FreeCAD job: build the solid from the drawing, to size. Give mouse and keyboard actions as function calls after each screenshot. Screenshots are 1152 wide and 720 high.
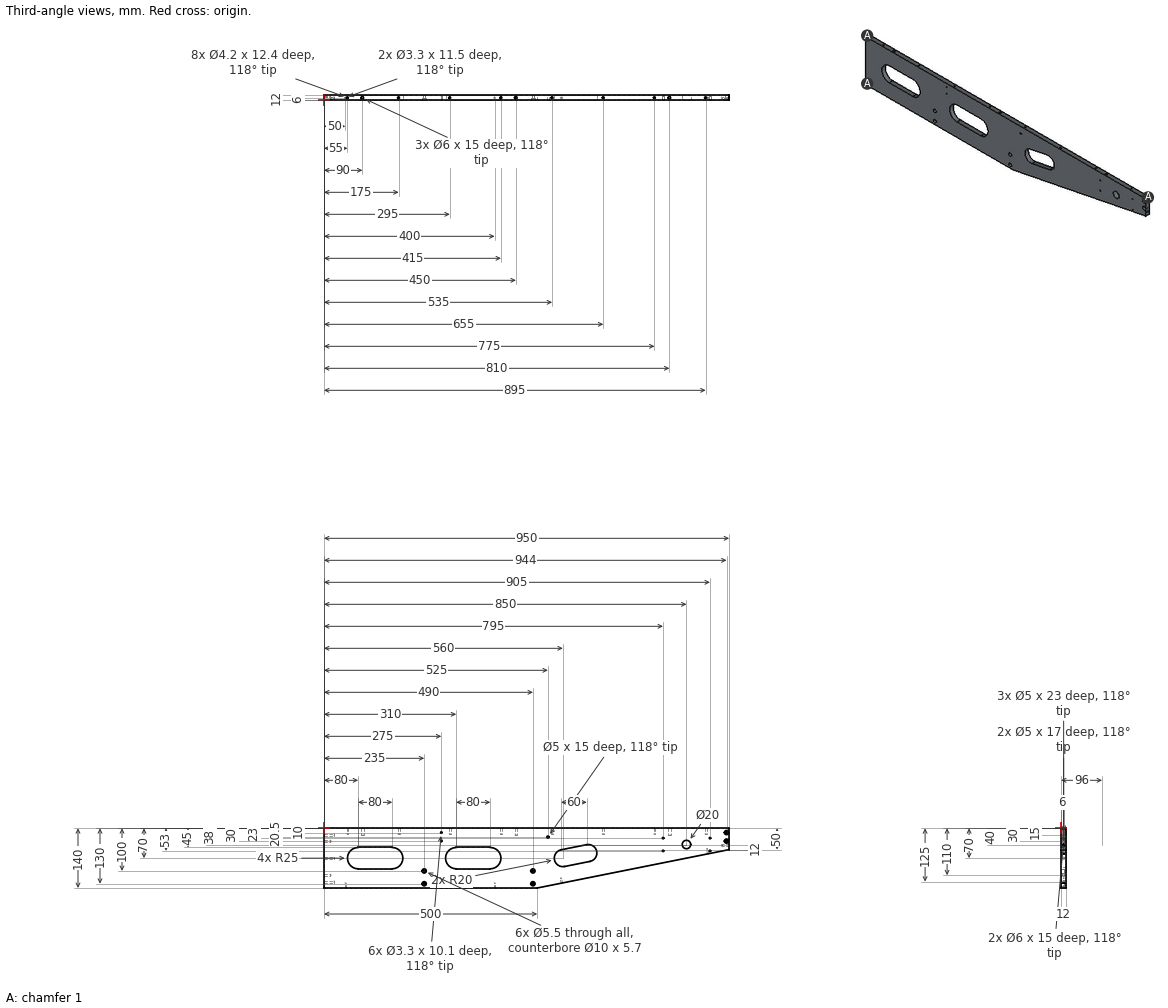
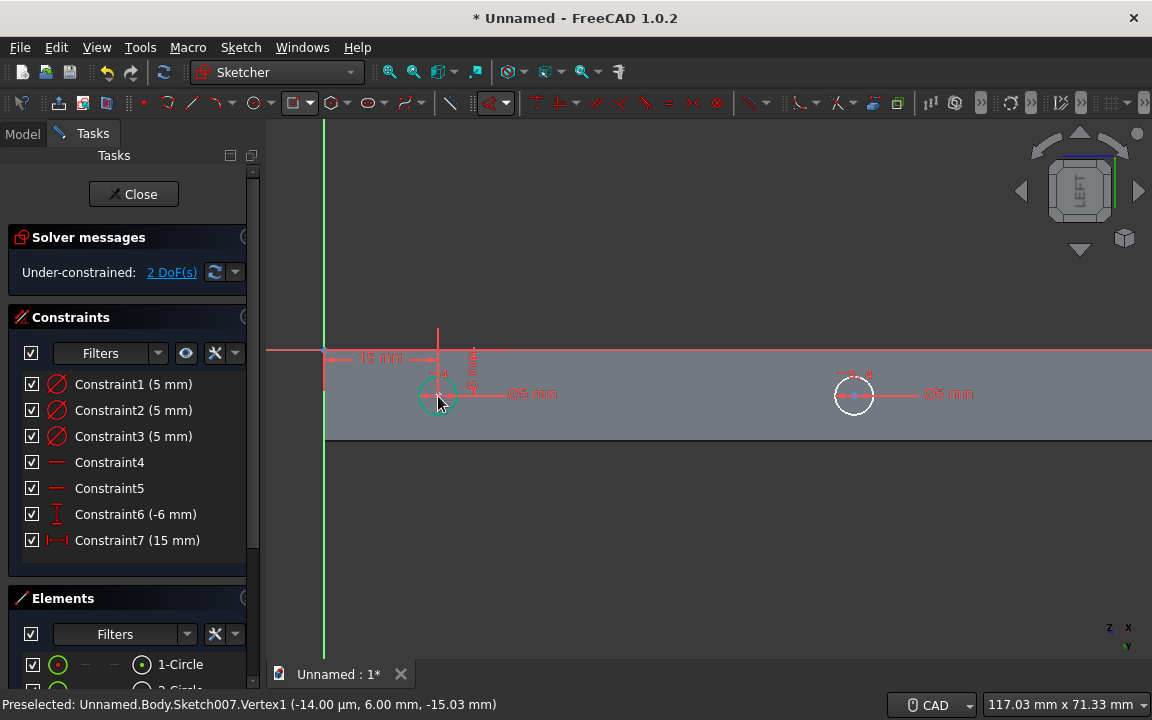
click(854, 396)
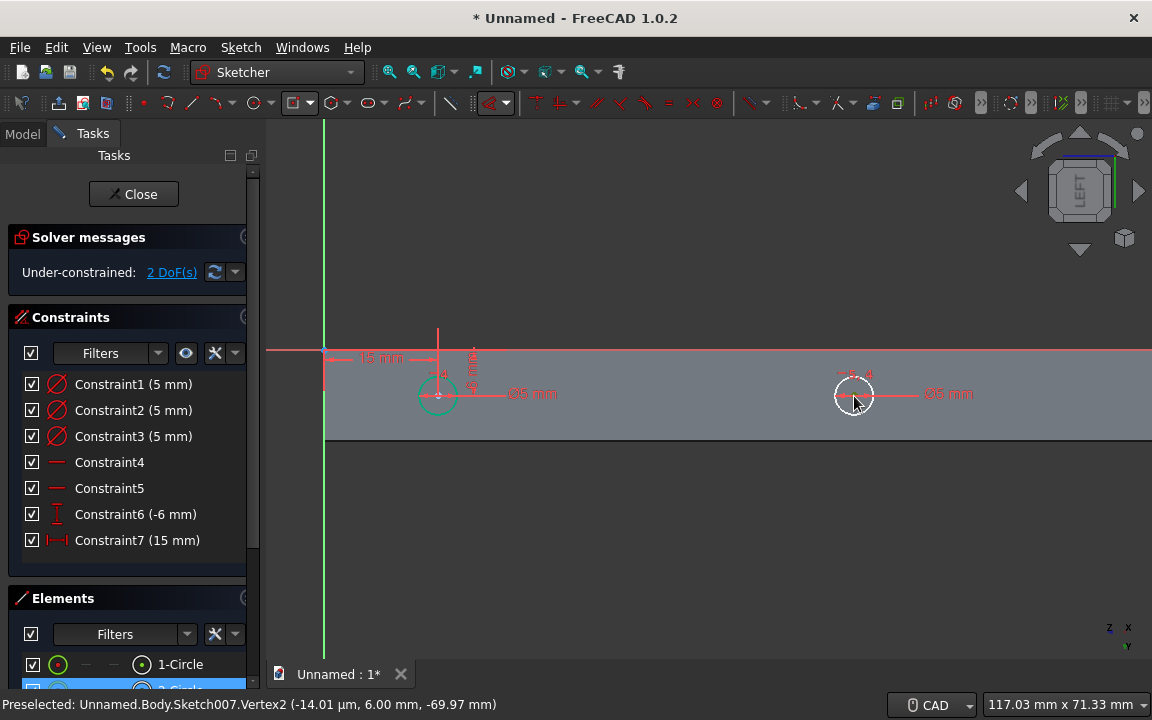
key(l)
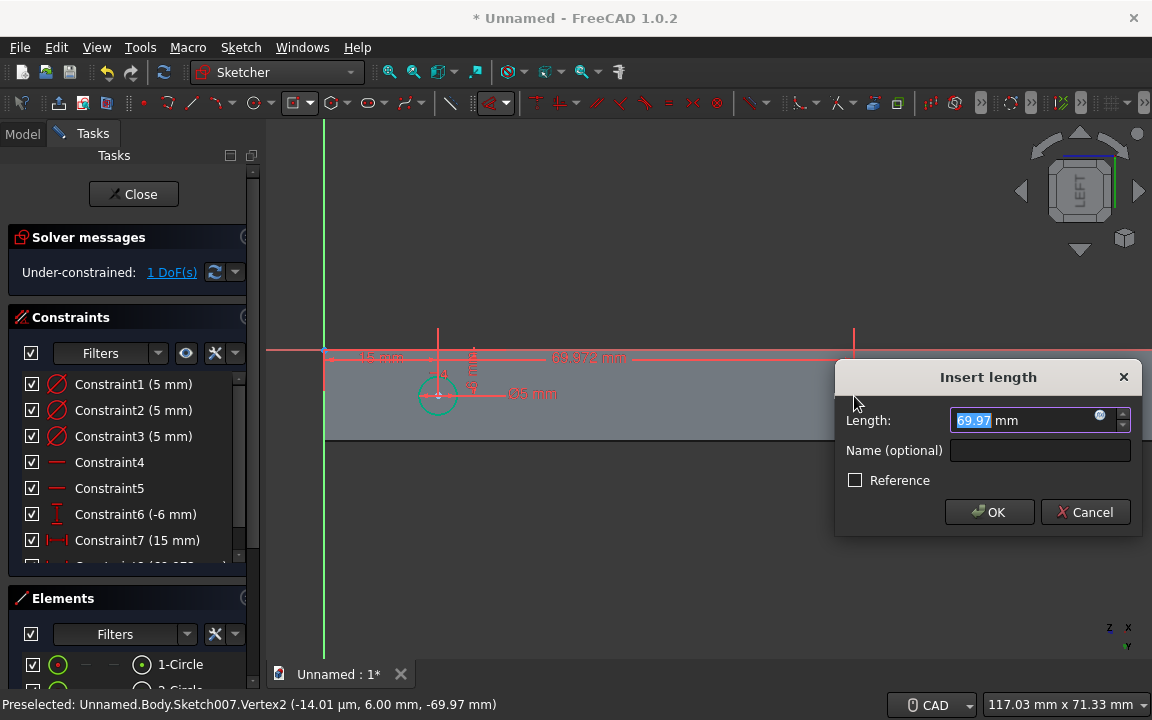
text(70)
key(Return)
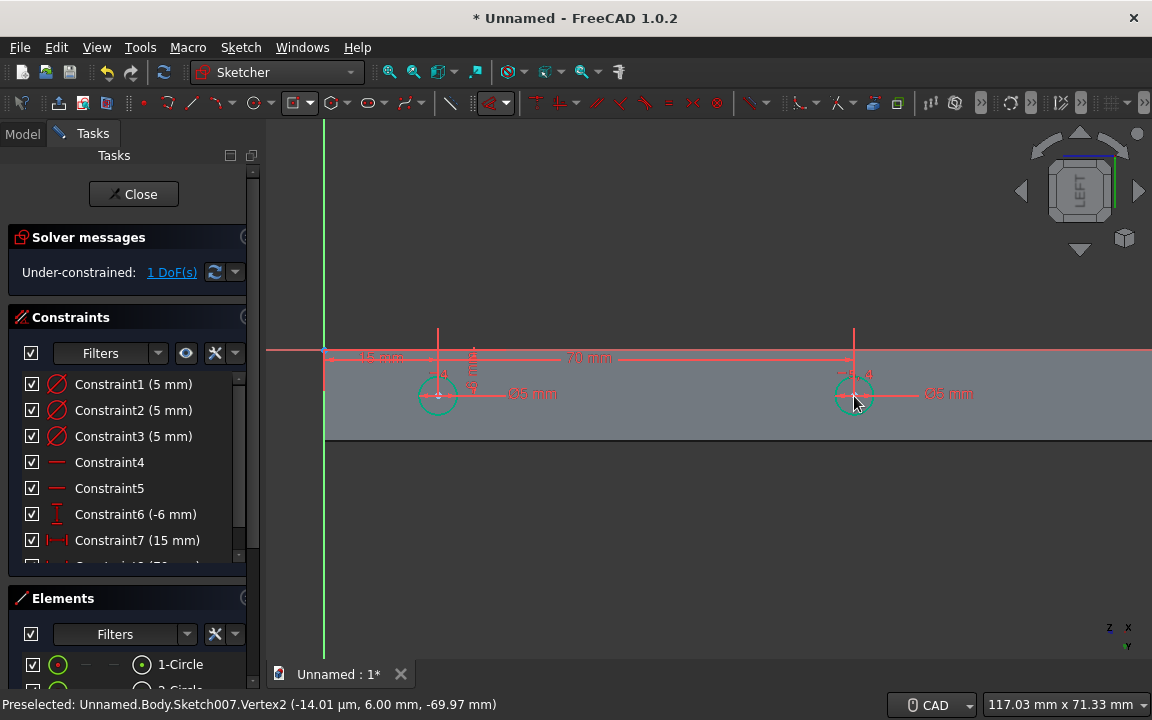
scroll(438, 397, down, 3)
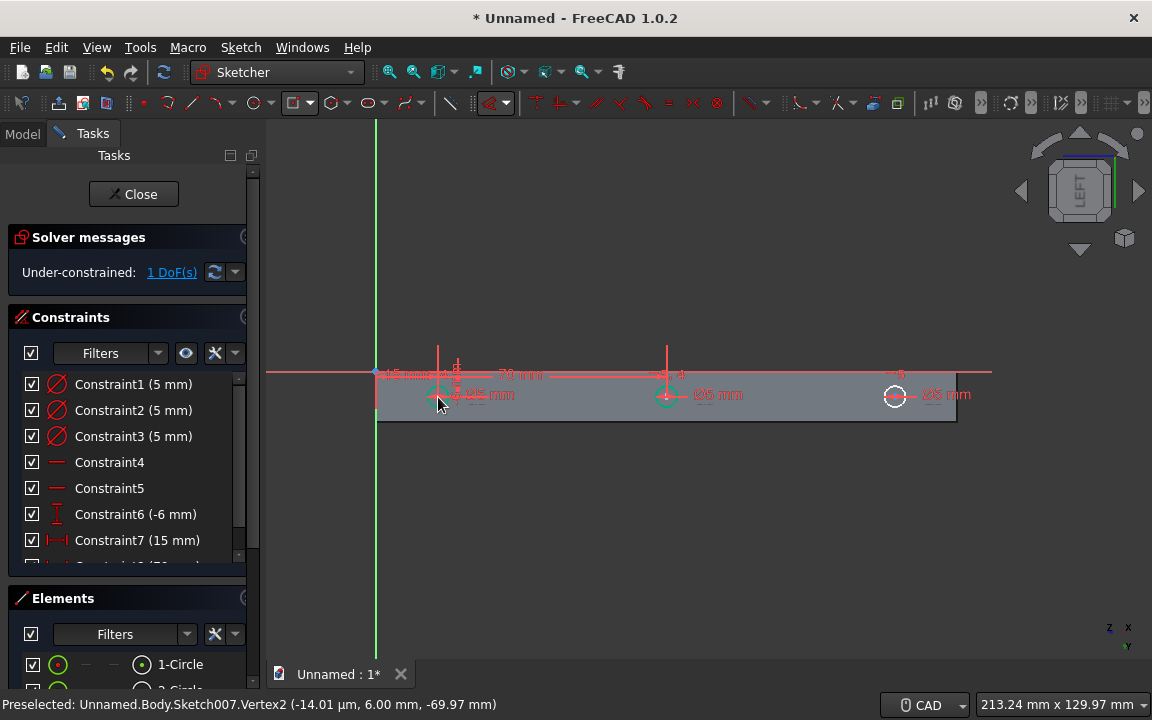
click(895, 397)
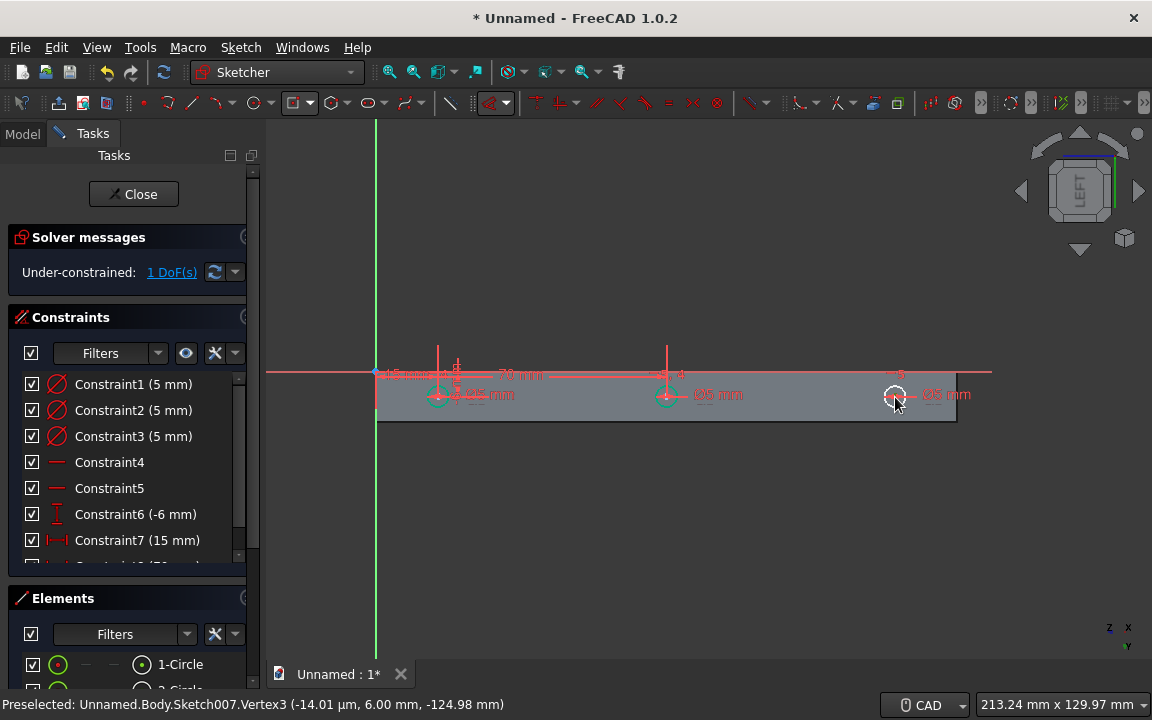
key(l)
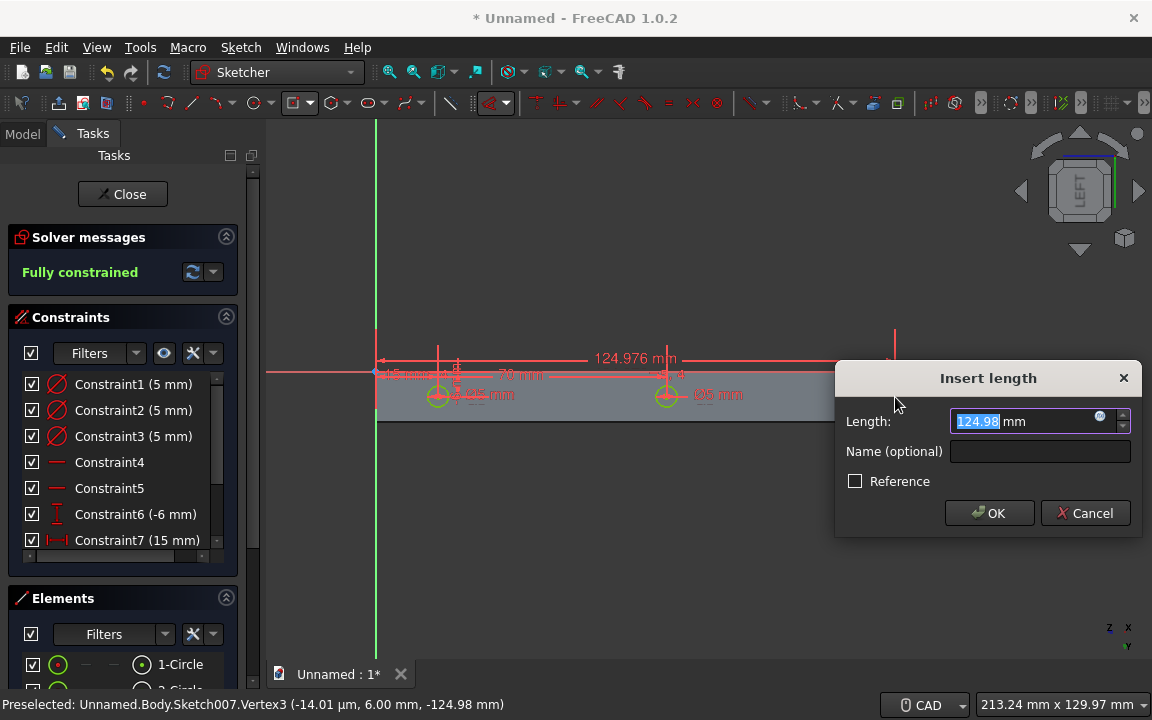
text(125)
key(Return)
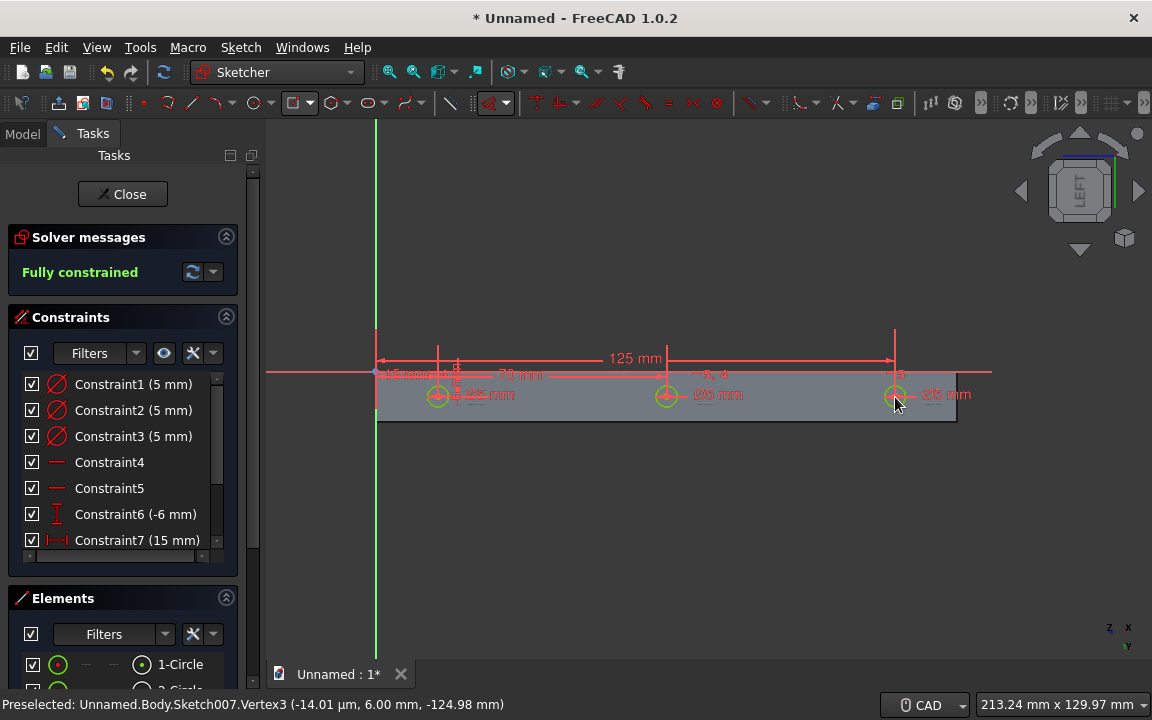
click(123, 194)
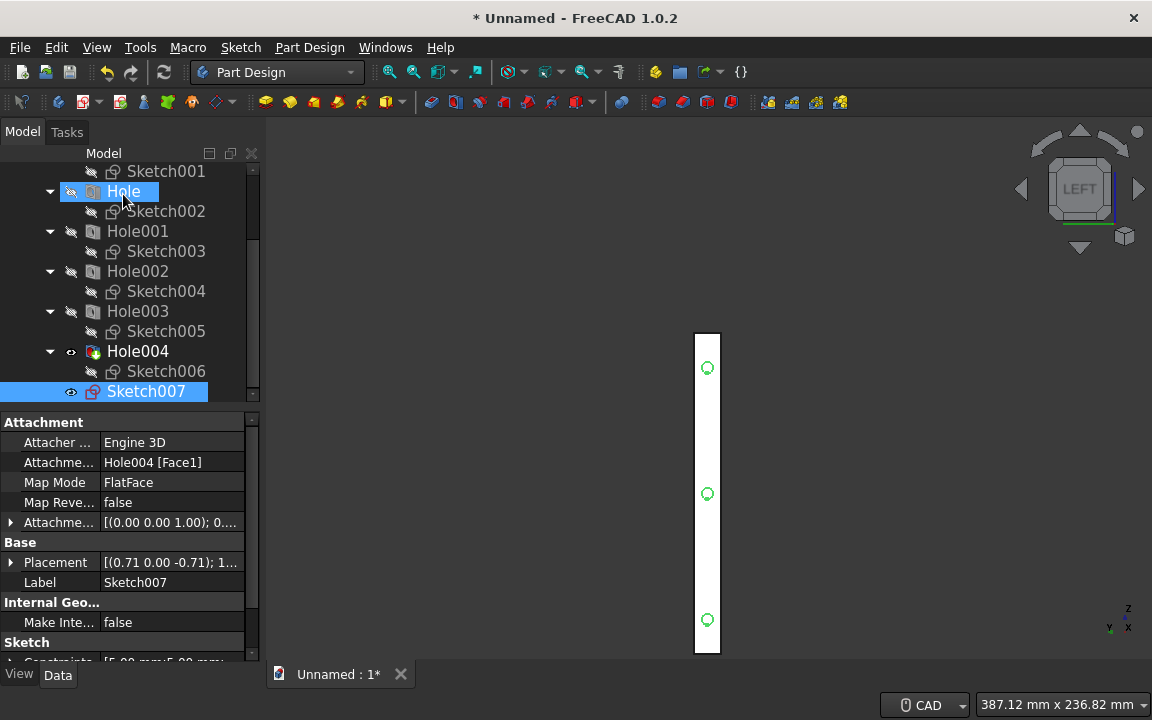
click(456, 102)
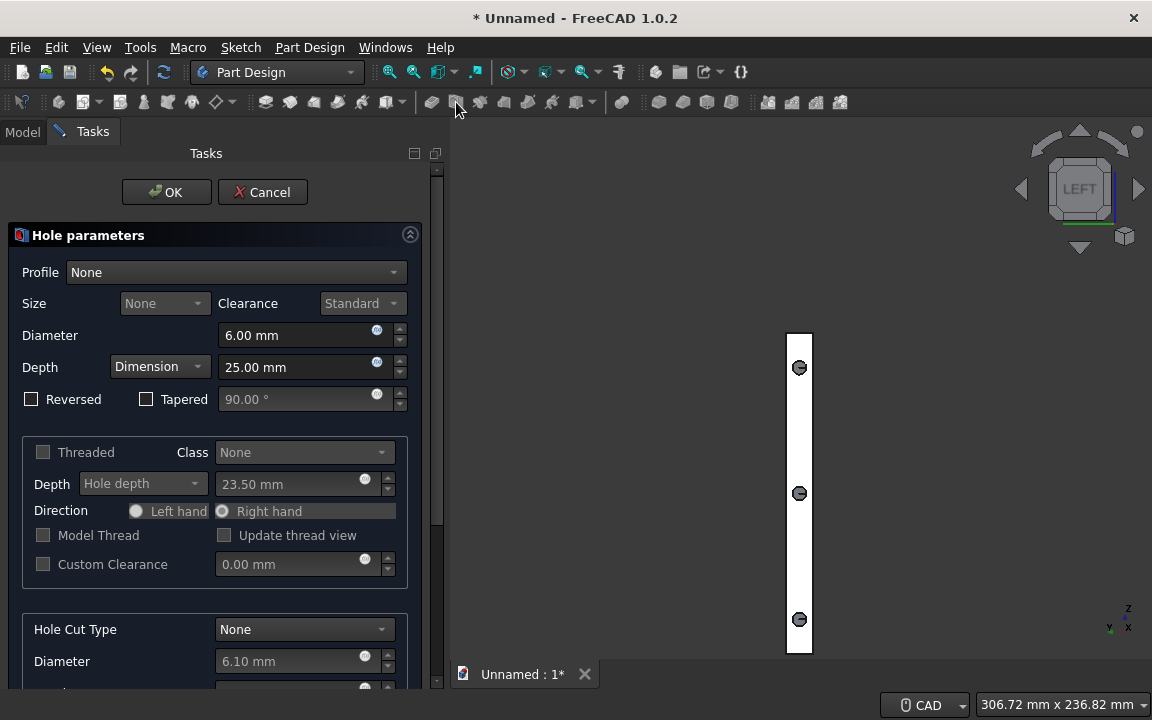
triple_click(305, 335)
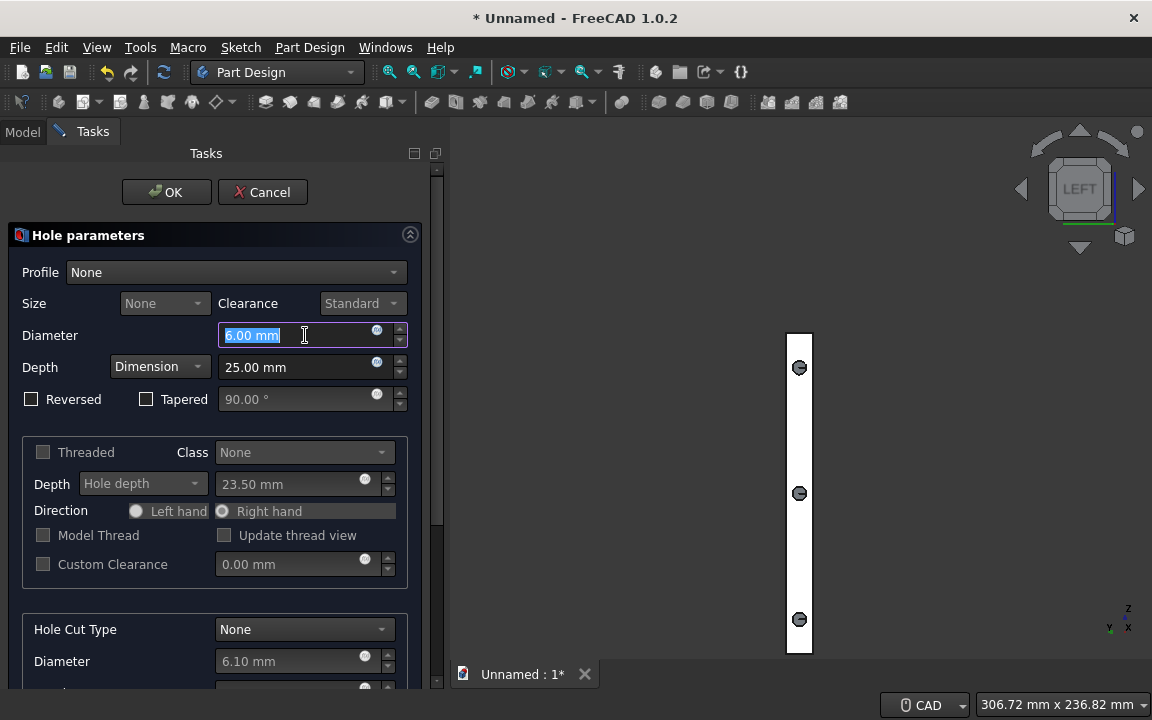
text(5)
key(Tab)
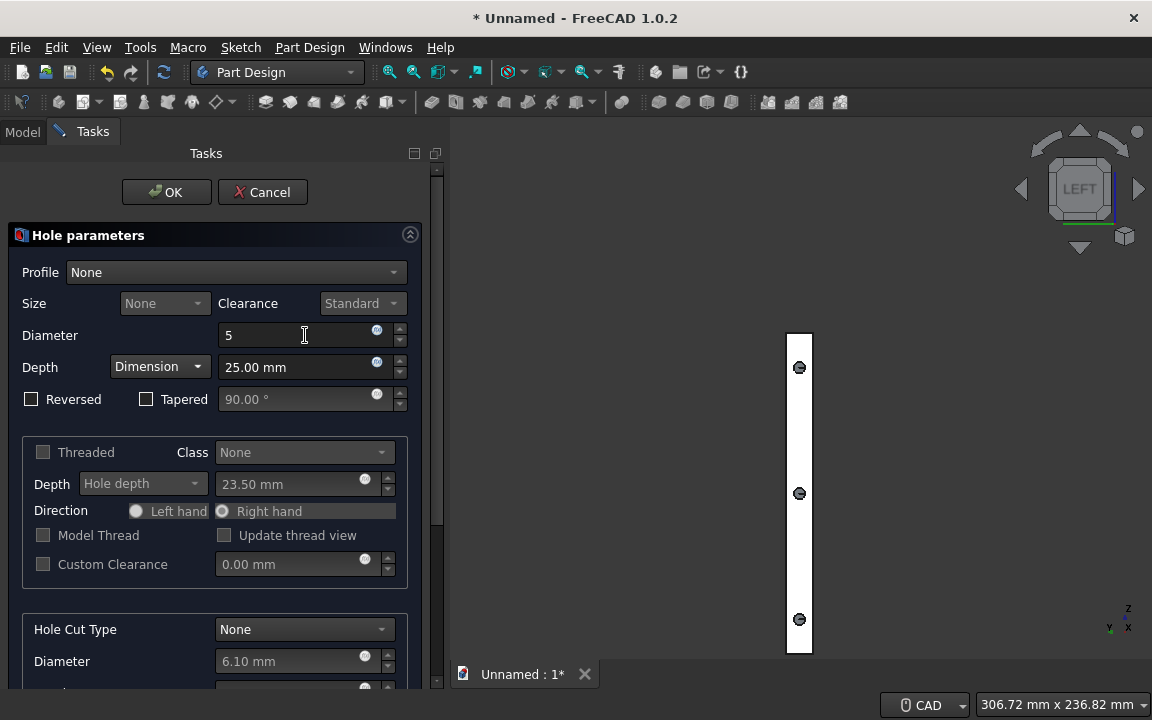
triple_click(305, 367)